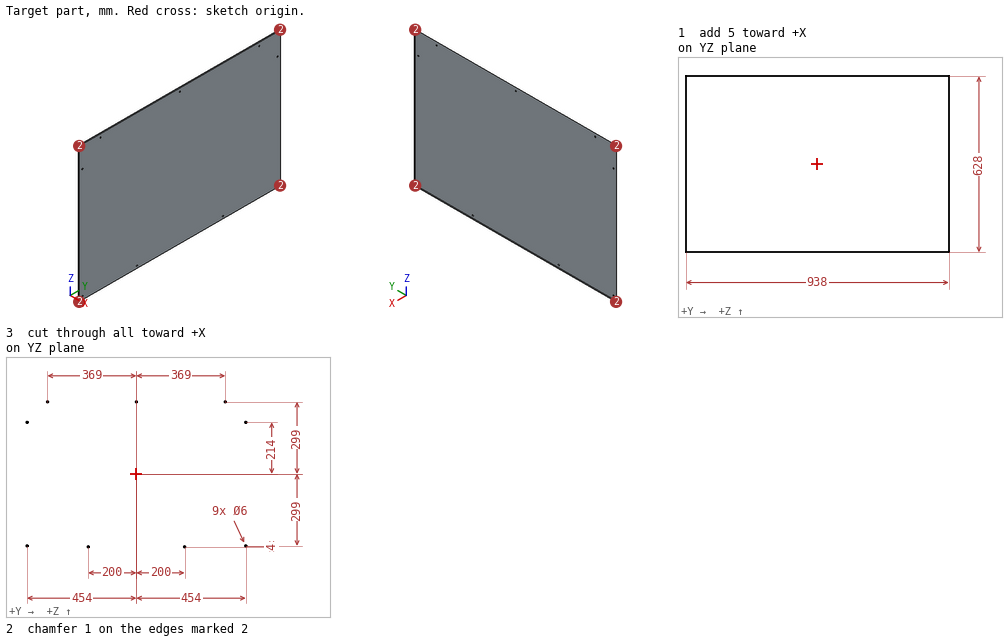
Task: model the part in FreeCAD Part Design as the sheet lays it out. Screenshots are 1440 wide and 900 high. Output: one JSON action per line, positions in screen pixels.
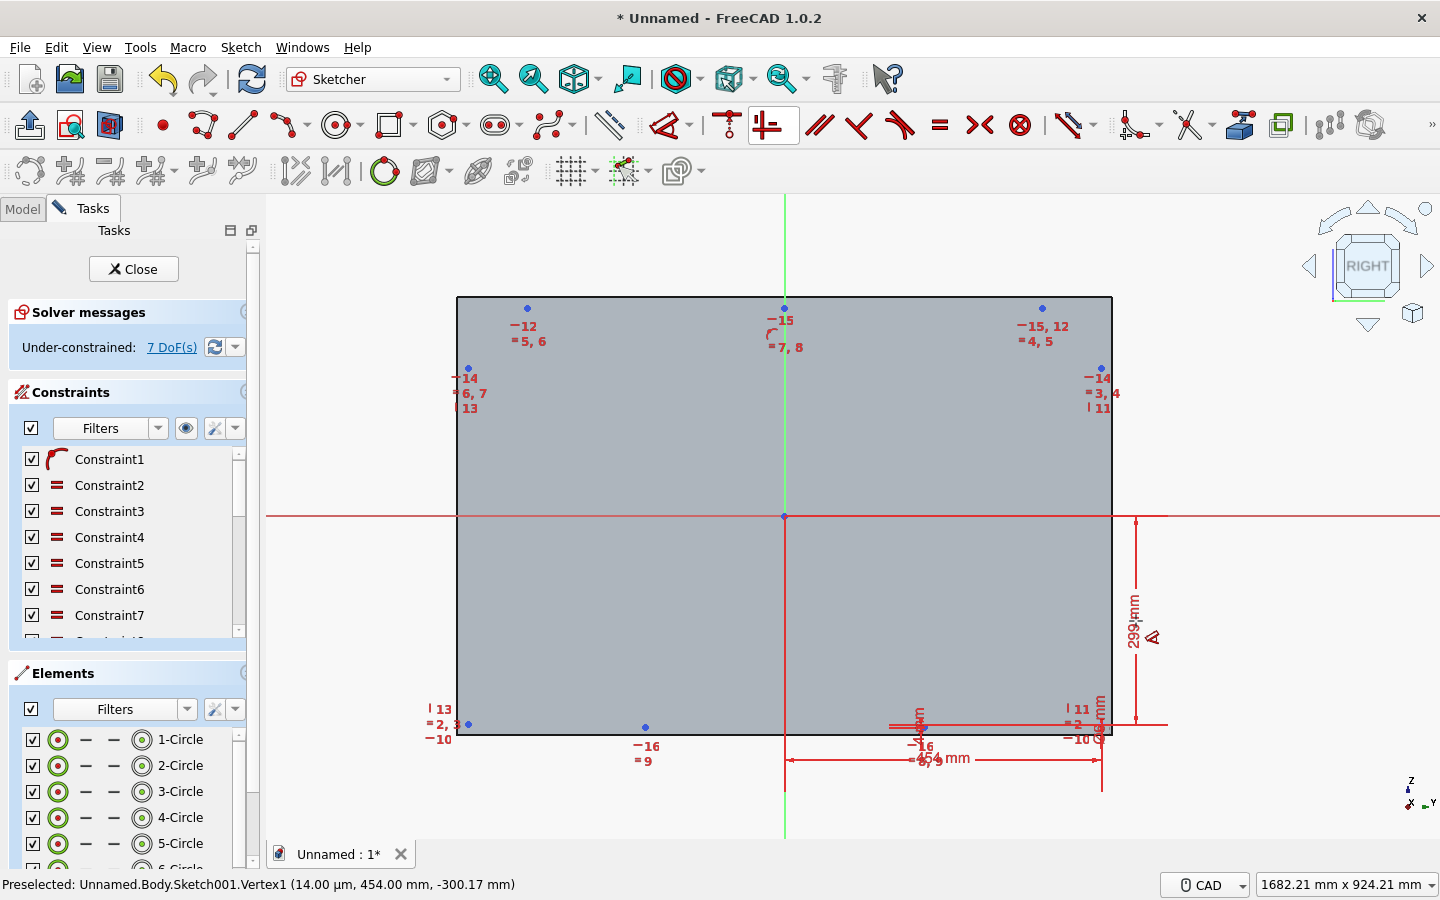
{"action": "left_click", "coordinate": [468, 725]}
{"action": "left_click", "coordinate": [626, 759]}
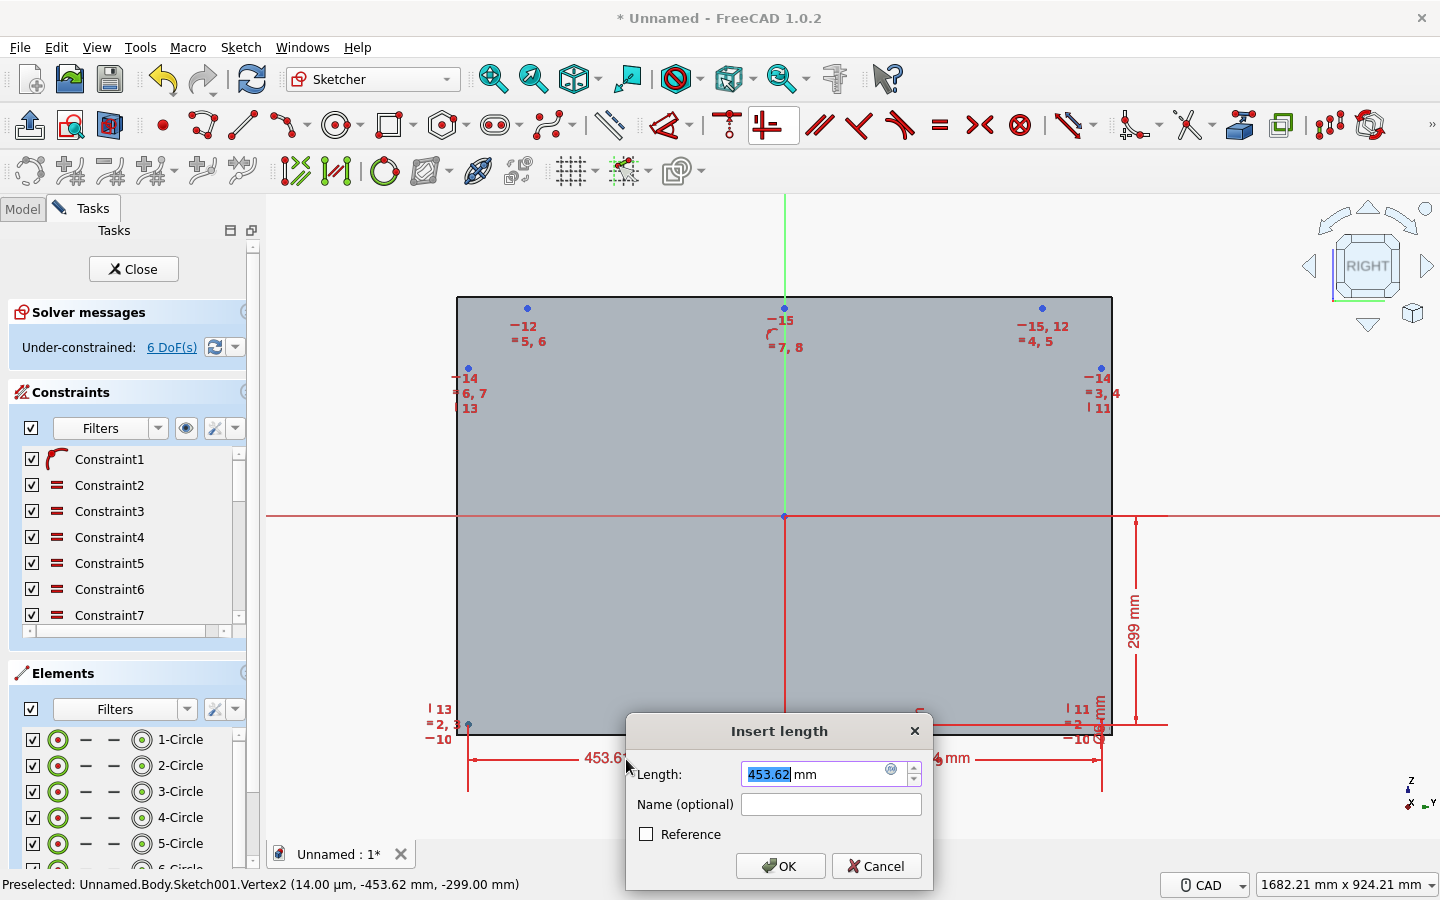
{"action": "type", "text": "454"}
{"action": "key", "text": "Return"}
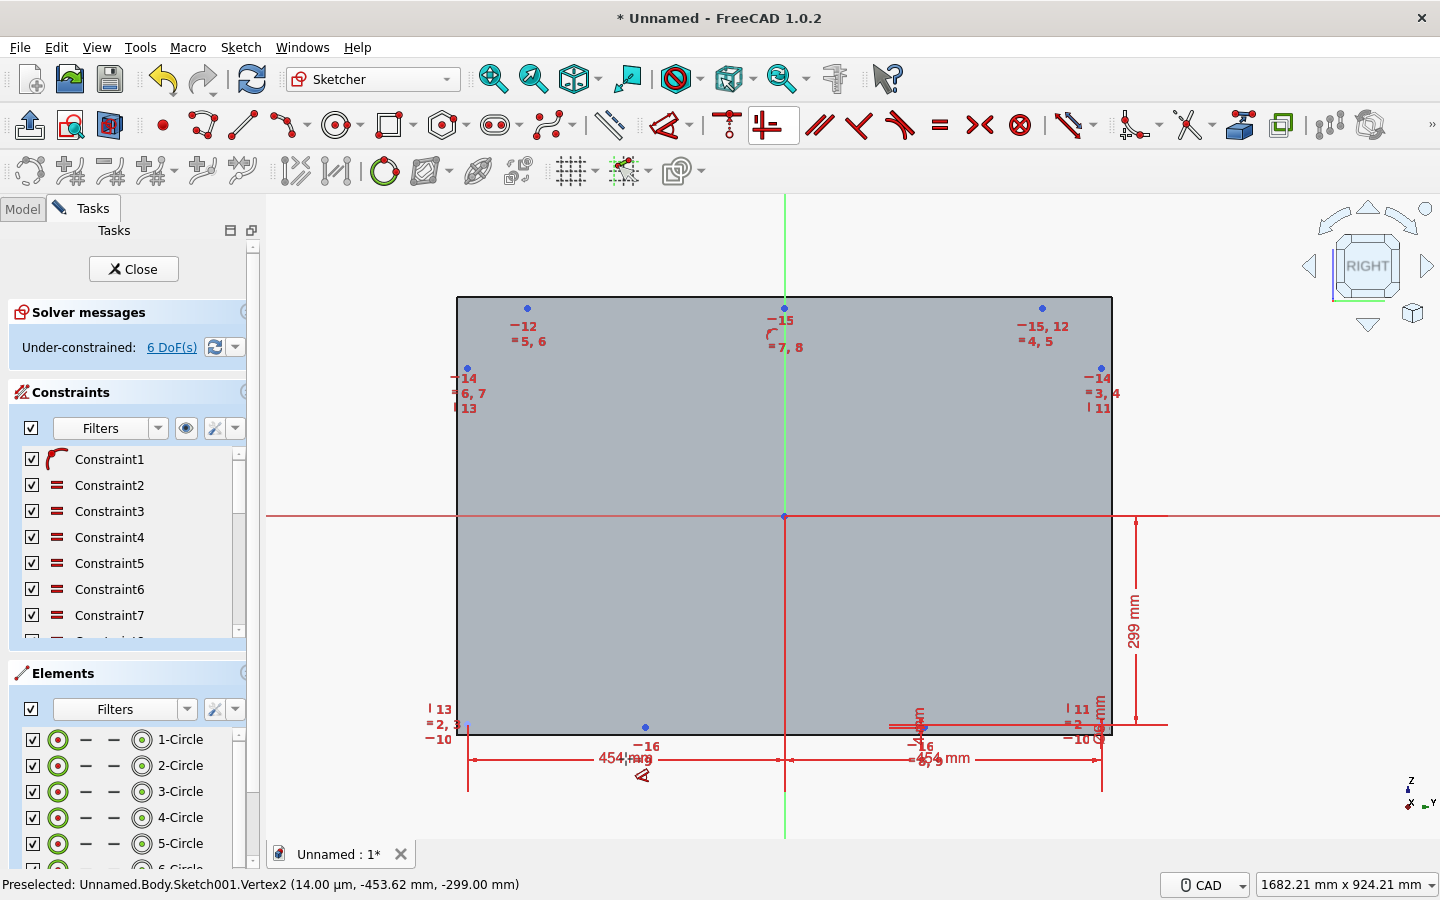
{"action": "left_click", "coordinate": [1102, 368]}
{"action": "left_click", "coordinate": [1136, 442]}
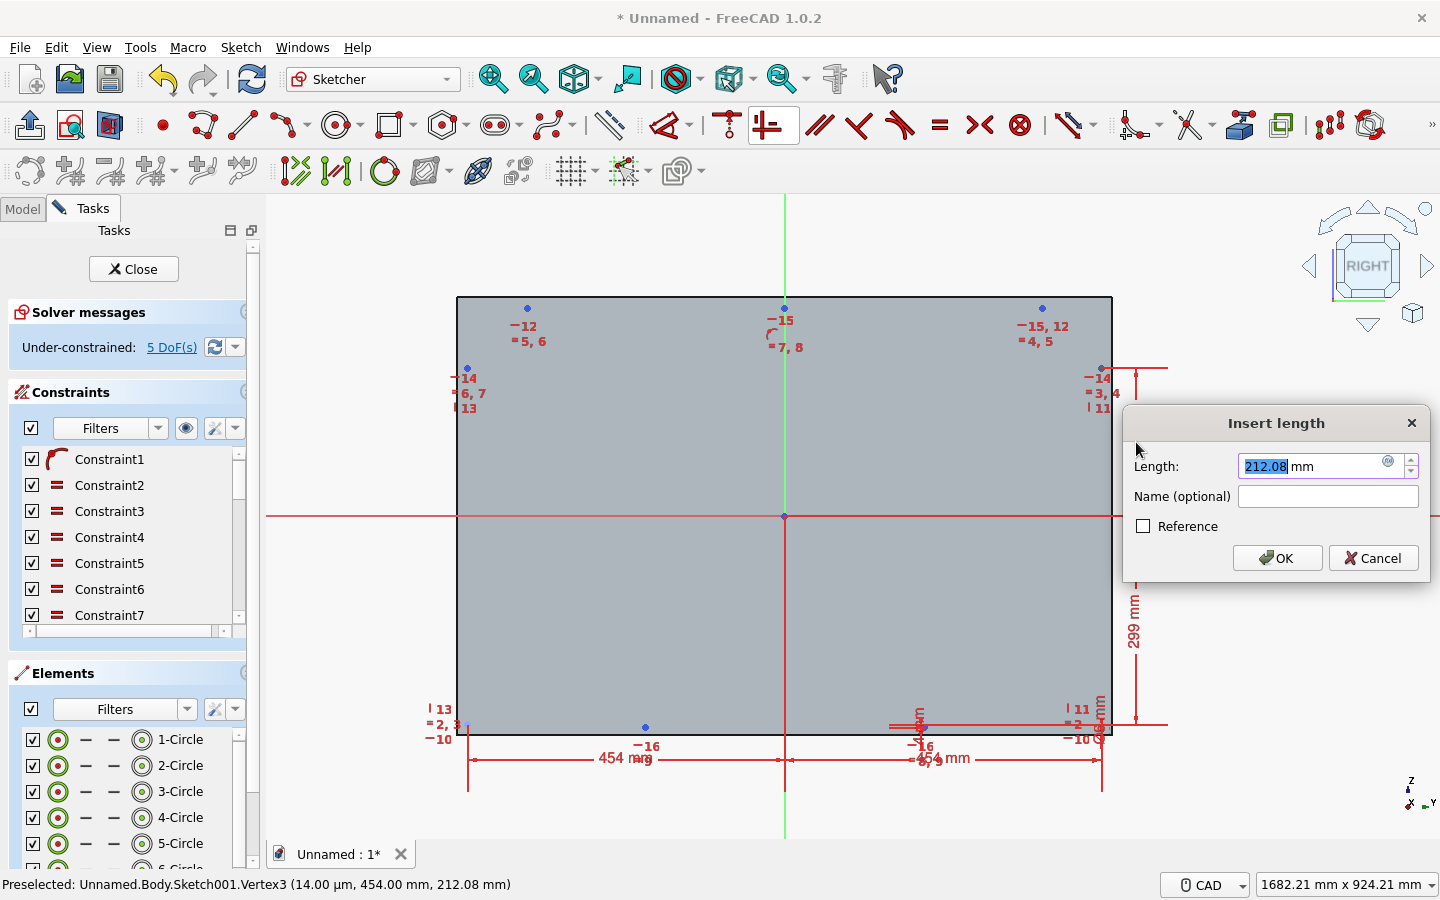
{"action": "type", "text": "214"}
{"action": "key", "text": "Return"}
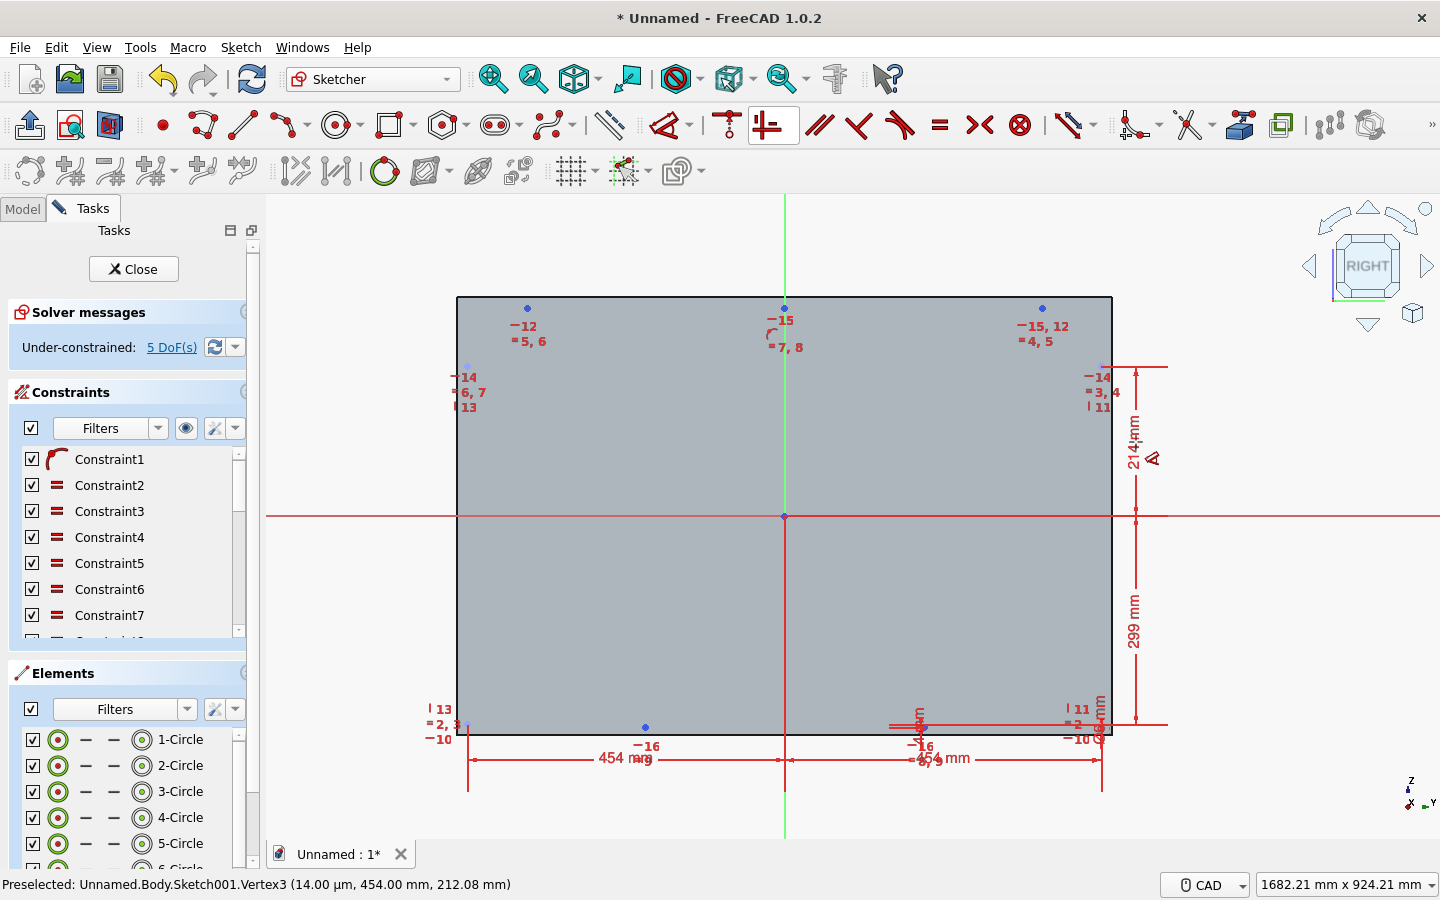
{"action": "left_click", "coordinate": [1042, 308]}
{"action": "left_click", "coordinate": [914, 274]}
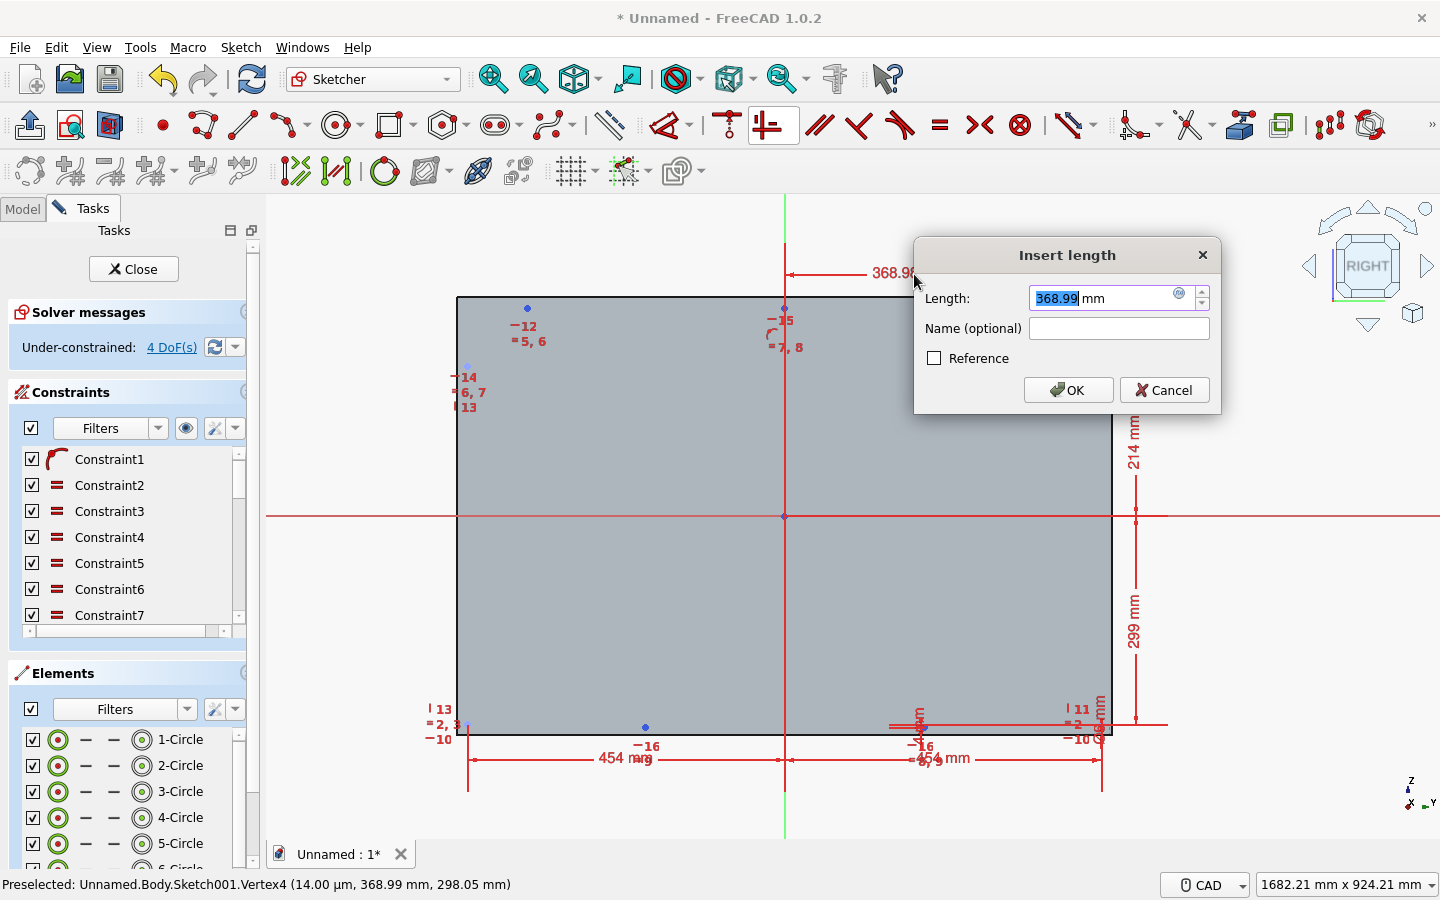
{"action": "type", "text": "369"}
{"action": "key", "text": "Return"}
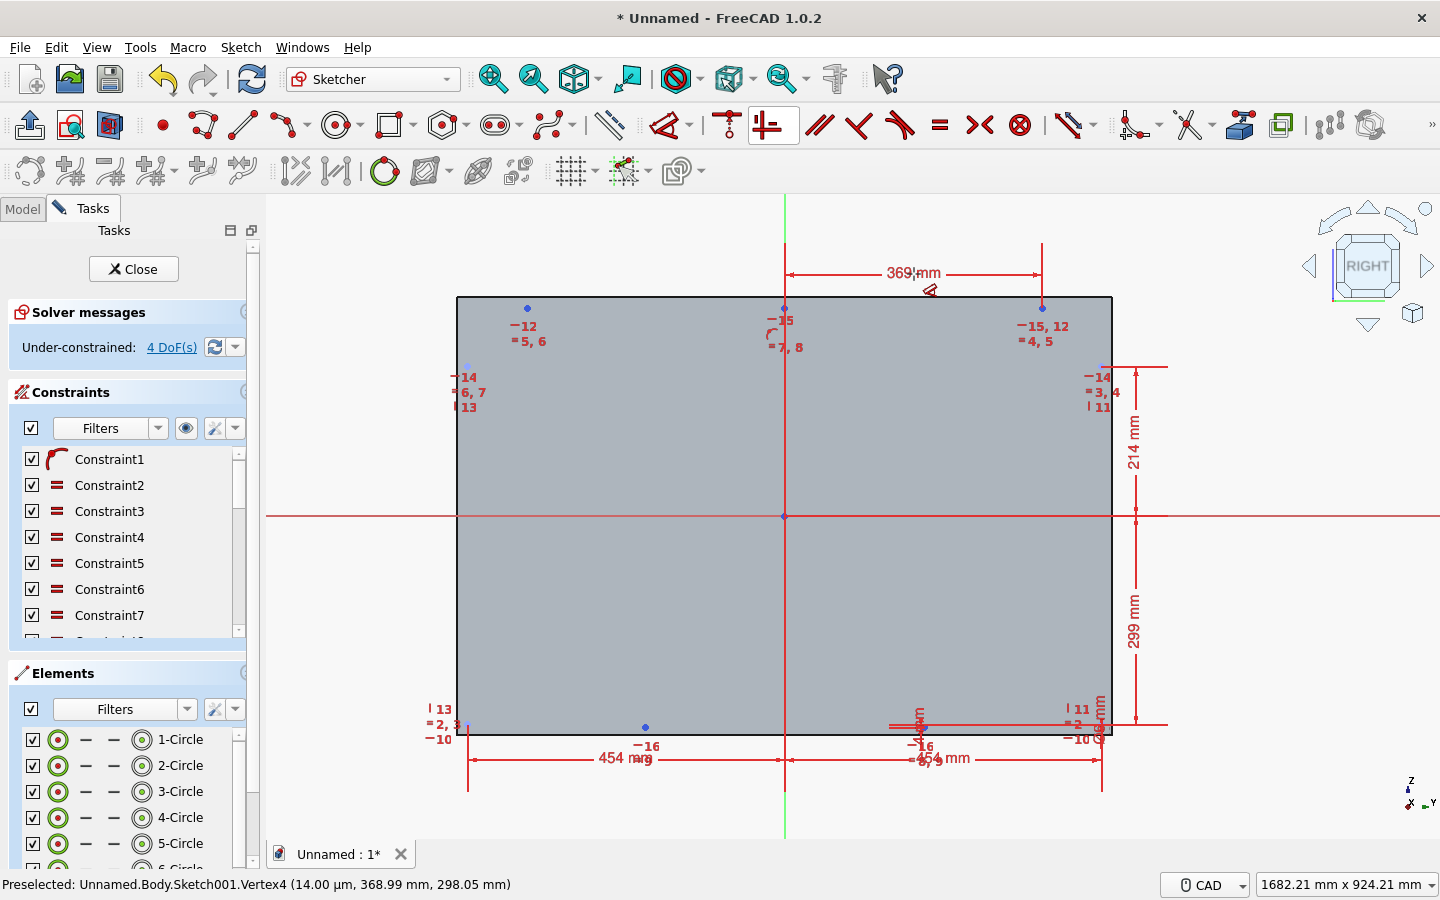
{"action": "left_click", "coordinate": [1042, 308]}
{"action": "left_click", "coordinate": [1076, 412]}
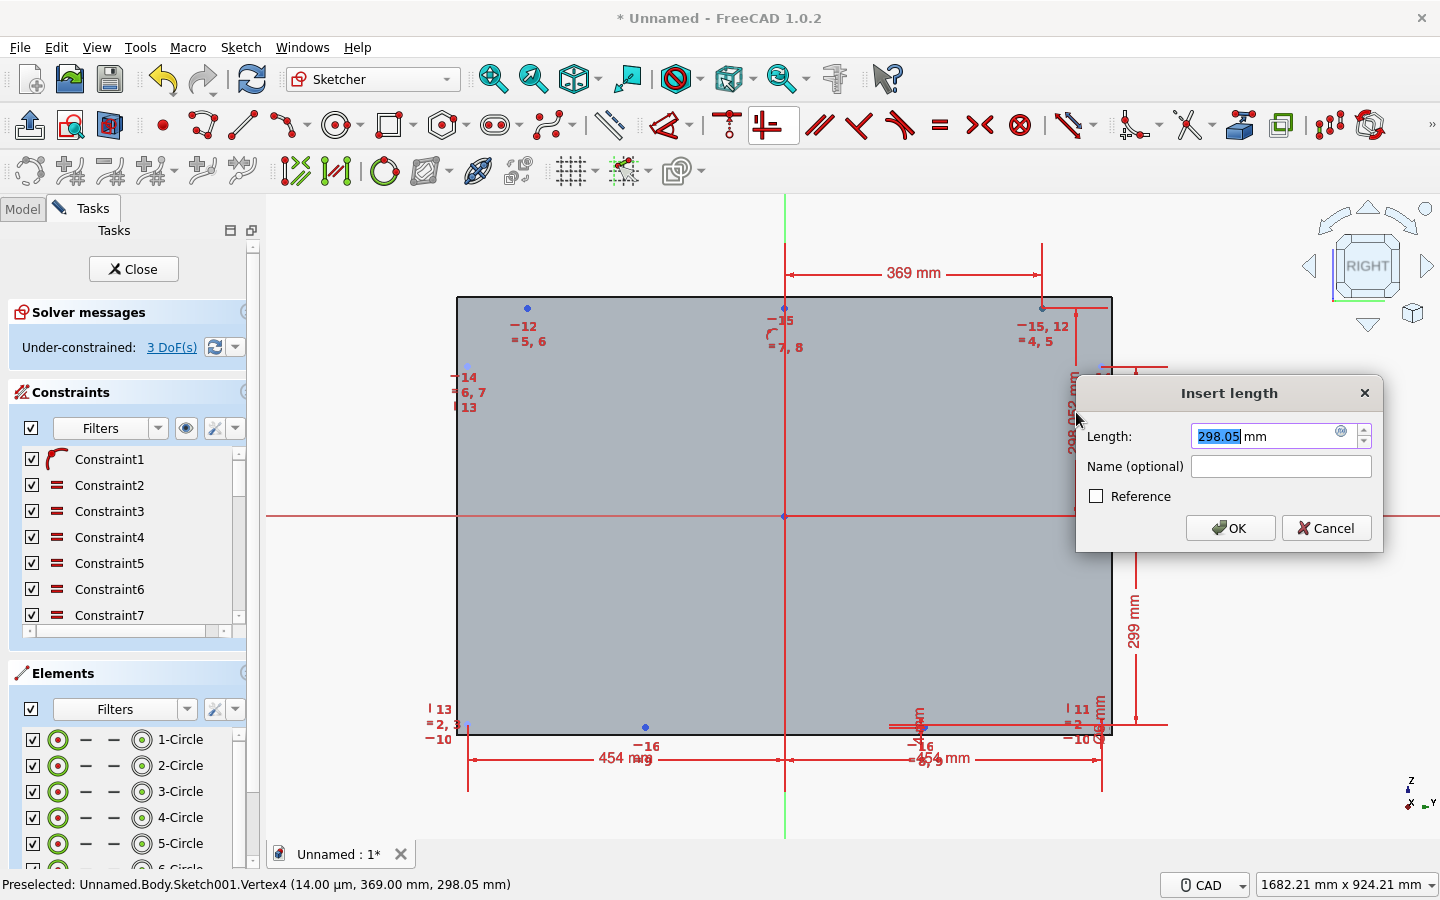
{"action": "type", "text": "299"}
{"action": "key", "text": "Return"}